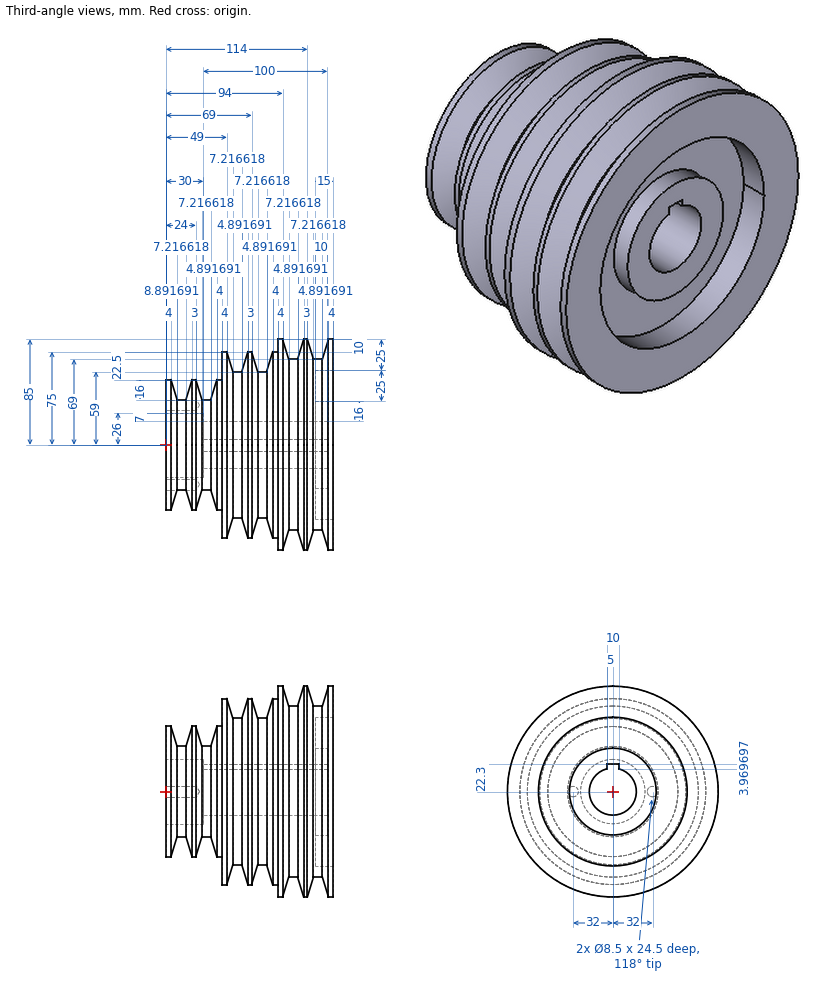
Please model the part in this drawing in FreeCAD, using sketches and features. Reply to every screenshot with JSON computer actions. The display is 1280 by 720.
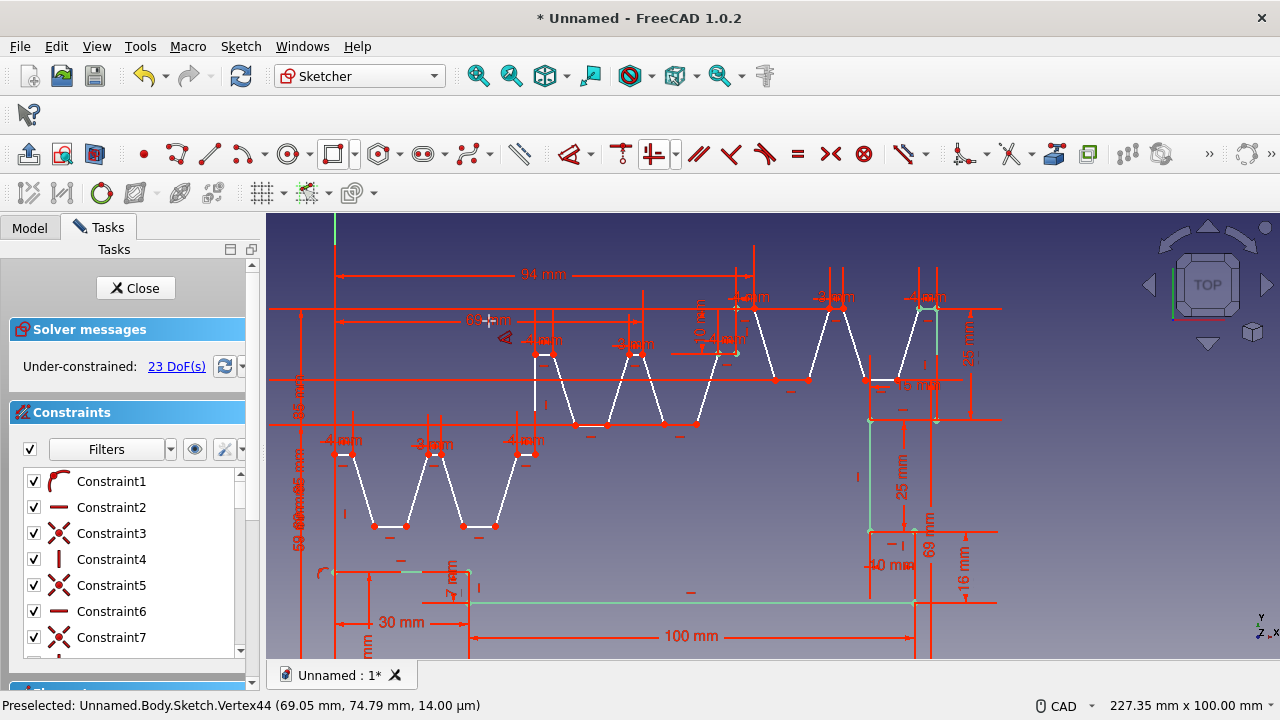
{"action": "left_click", "coordinate": [643, 355]}
{"action": "left_click", "coordinate": [301, 556]}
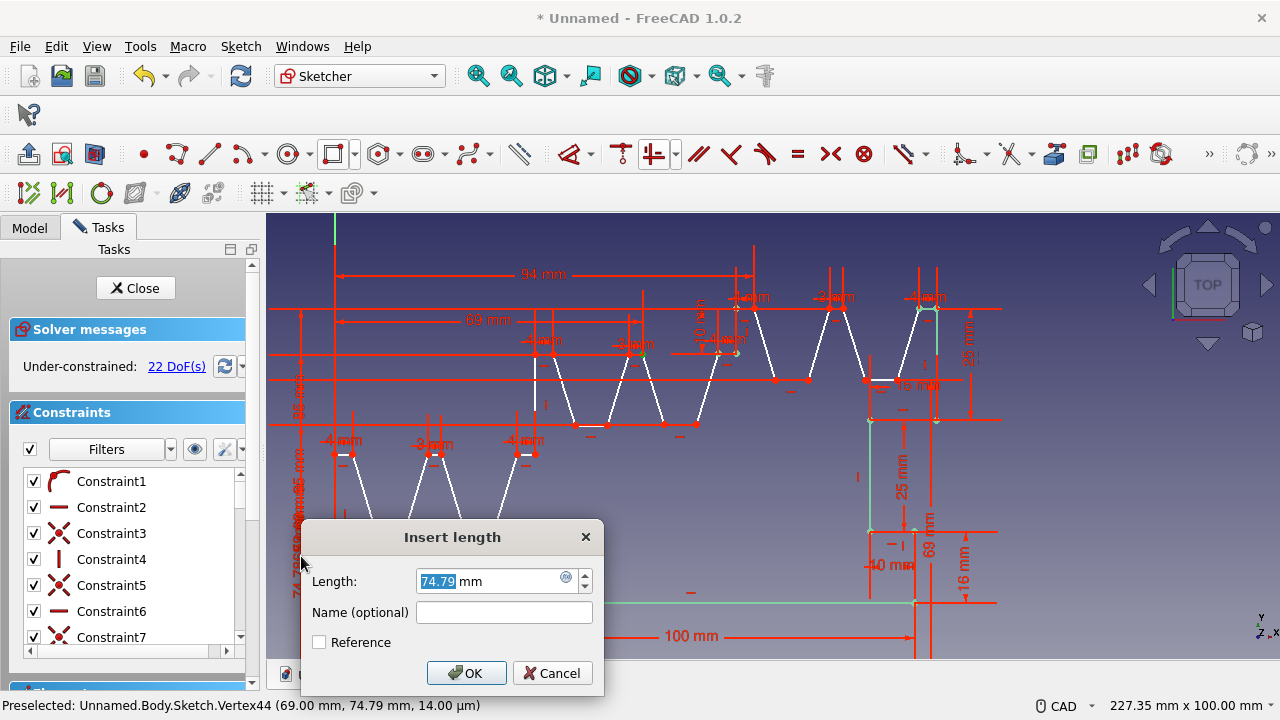
{"action": "type", "text": "75"}
{"action": "key", "text": "Return"}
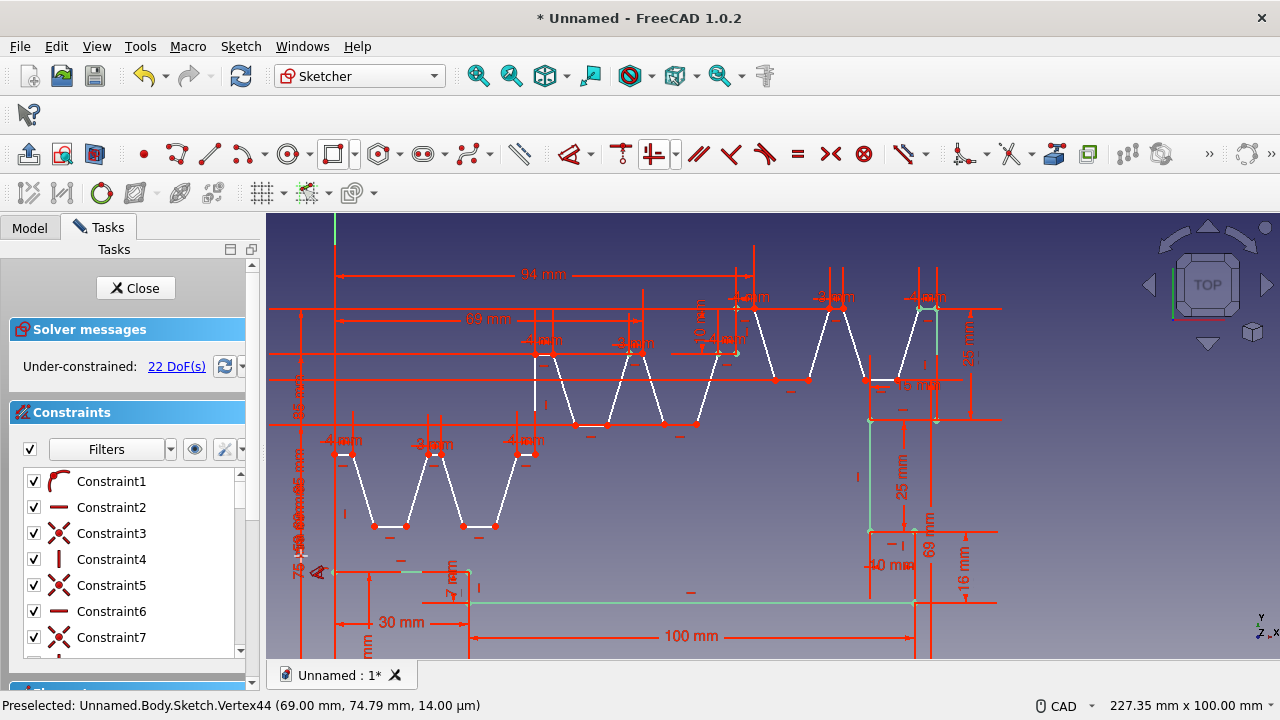
{"action": "left_click", "coordinate": [607, 426]}
{"action": "left_click", "coordinate": [301, 600]}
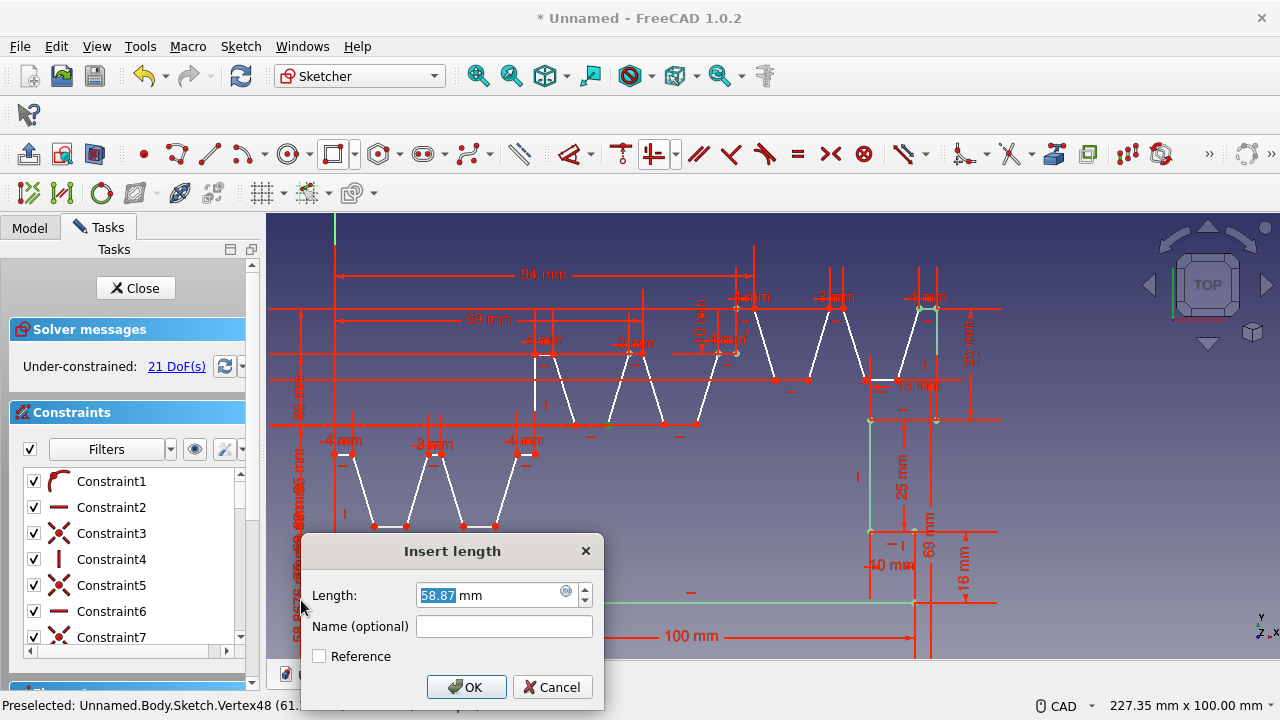
{"action": "type", "text": "59"}
{"action": "key", "text": "Return"}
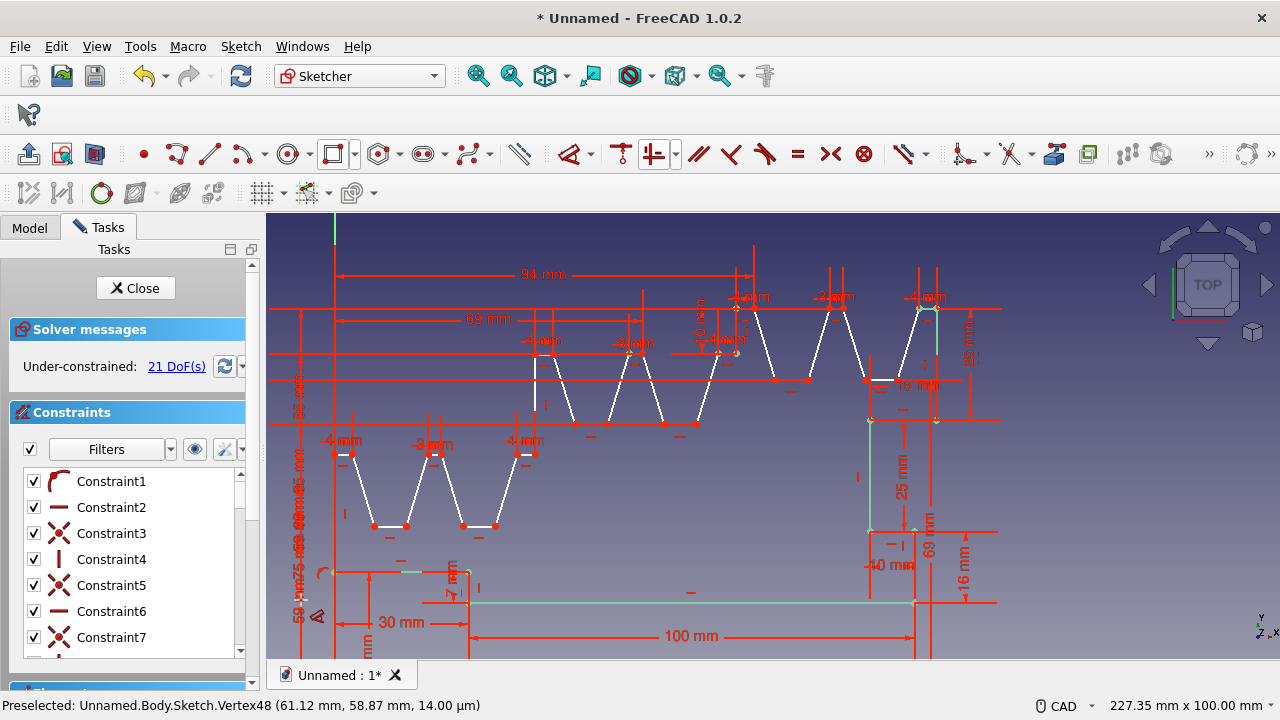
{"action": "left_click", "coordinate": [553, 355]}
{"action": "left_click", "coordinate": [394, 321]}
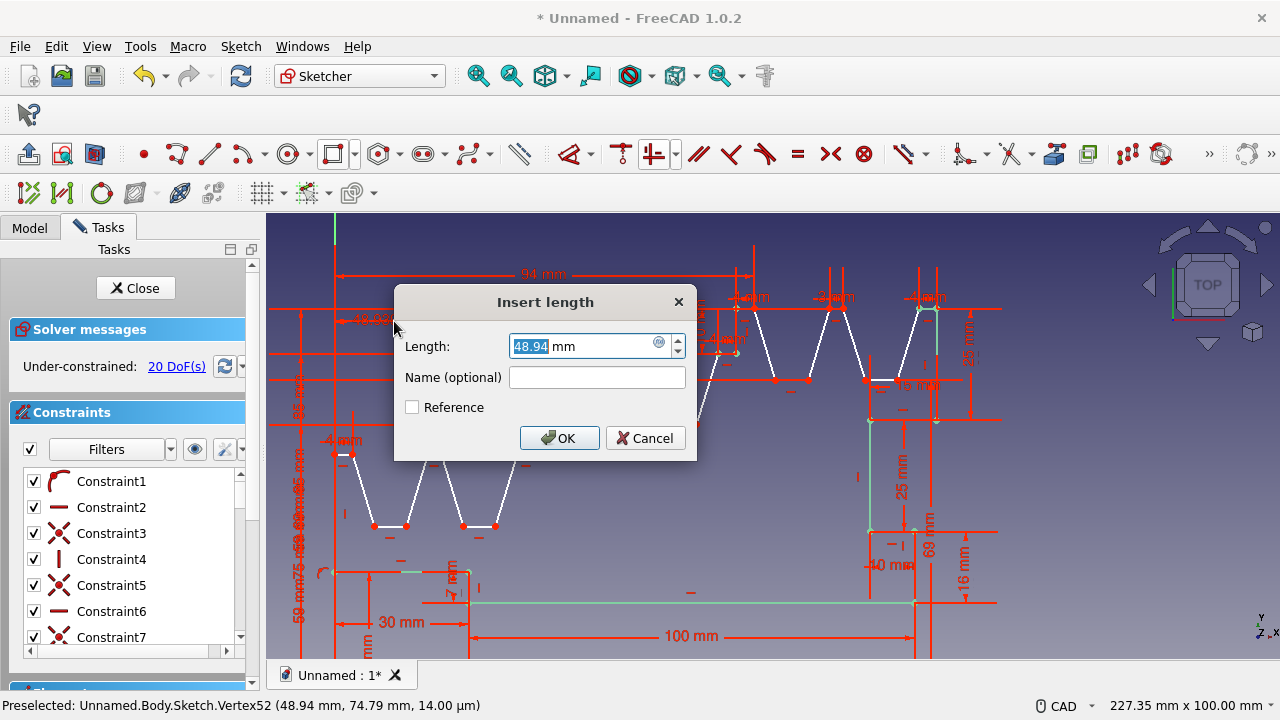
{"action": "type", "text": "49"}
{"action": "key", "text": "Return"}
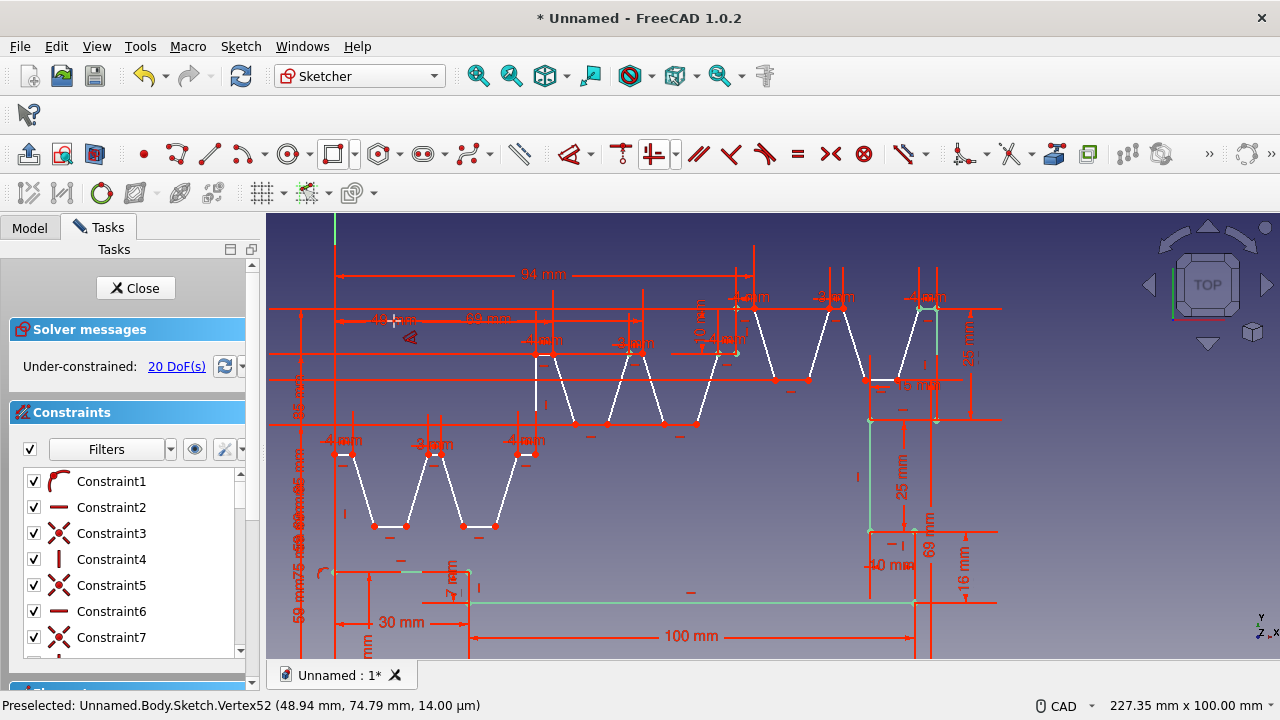
{"action": "left_click", "coordinate": [553, 355]}
{"action": "left_click", "coordinate": [587, 493]}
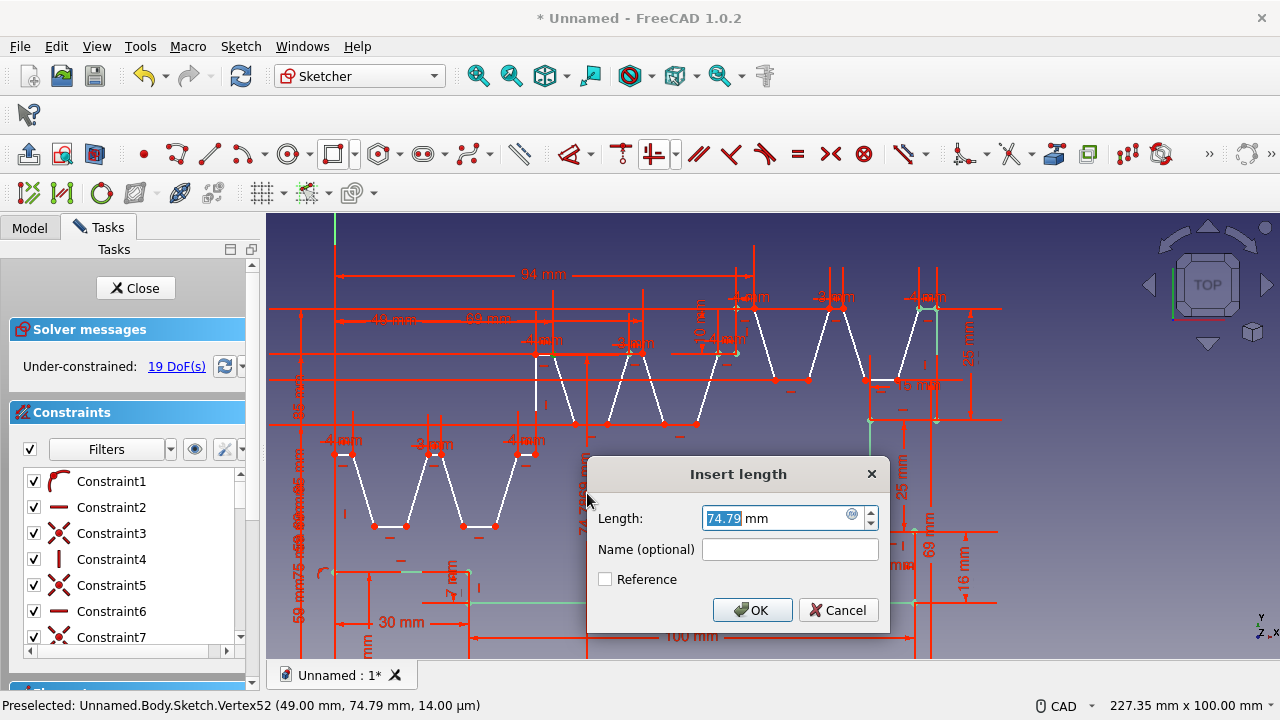
{"action": "type", "text": "75"}
{"action": "key", "text": "Return"}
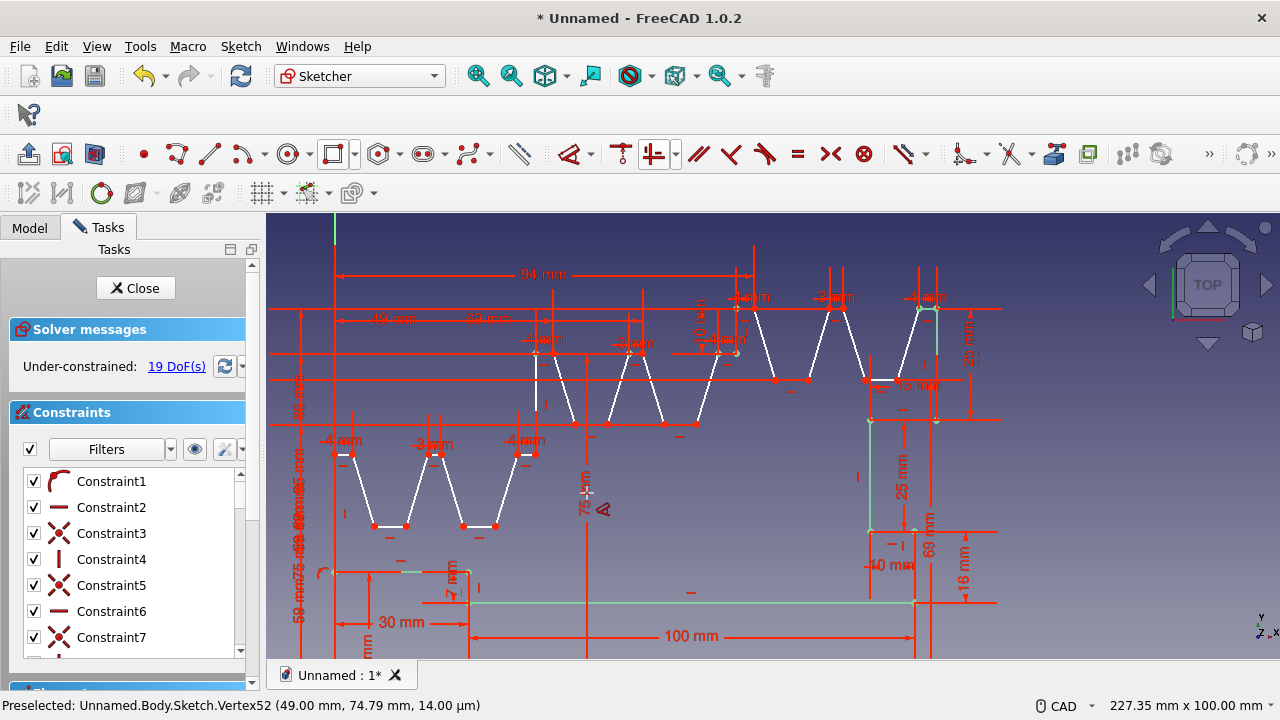
{"action": "left_click", "coordinate": [441, 455]}
{"action": "left_click", "coordinate": [388, 421]}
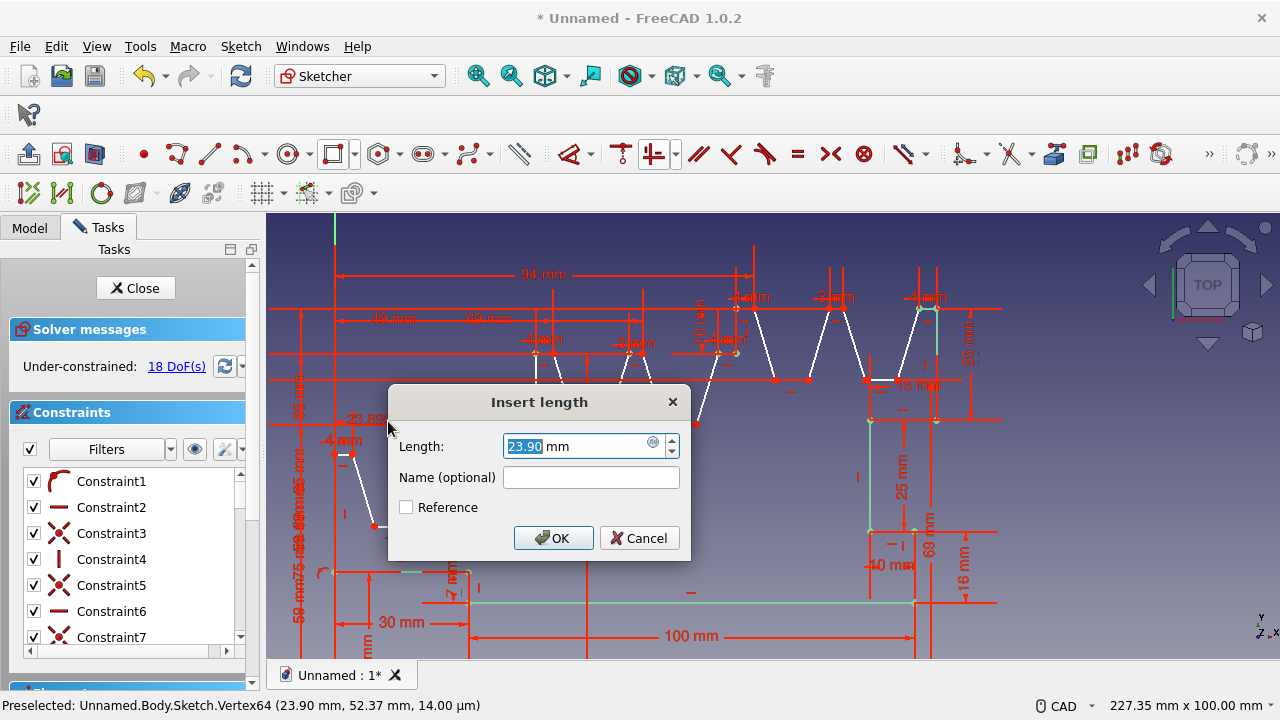
{"action": "type", "text": "24"}
{"action": "key", "text": "Return"}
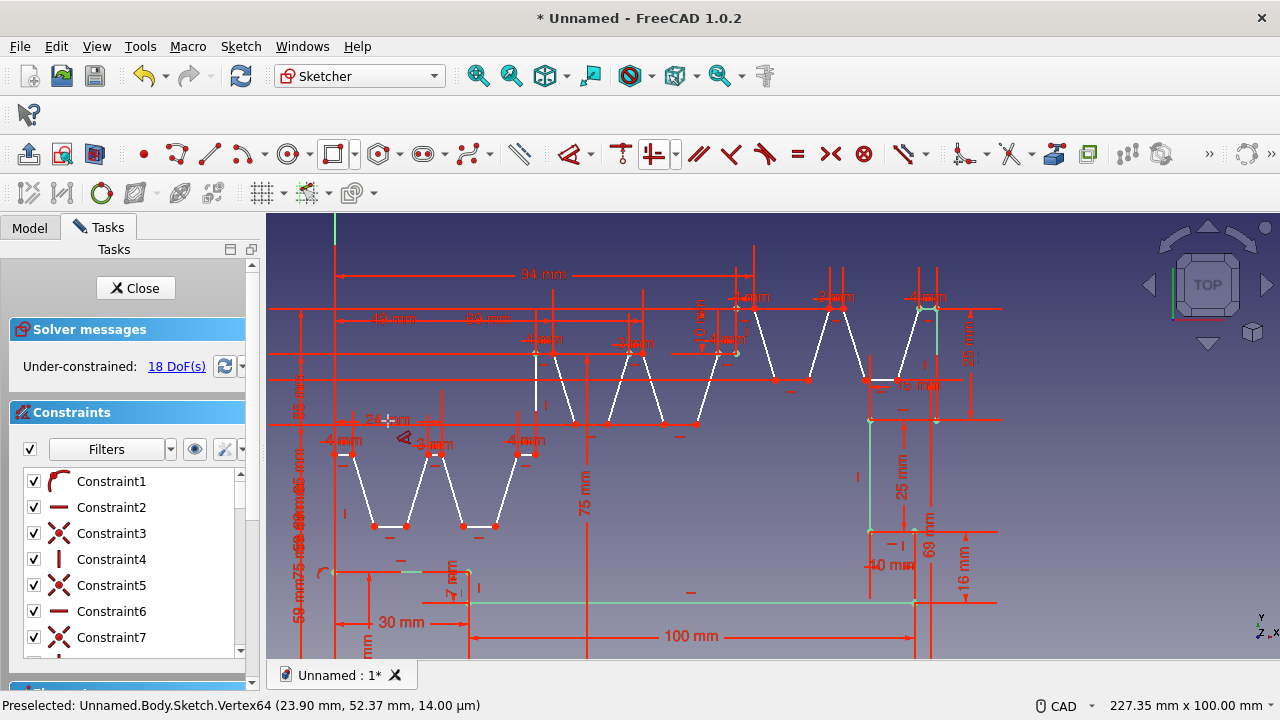
{"action": "left_click", "coordinate": [511, 476]}
{"action": "left_click", "coordinate": [461, 474]}